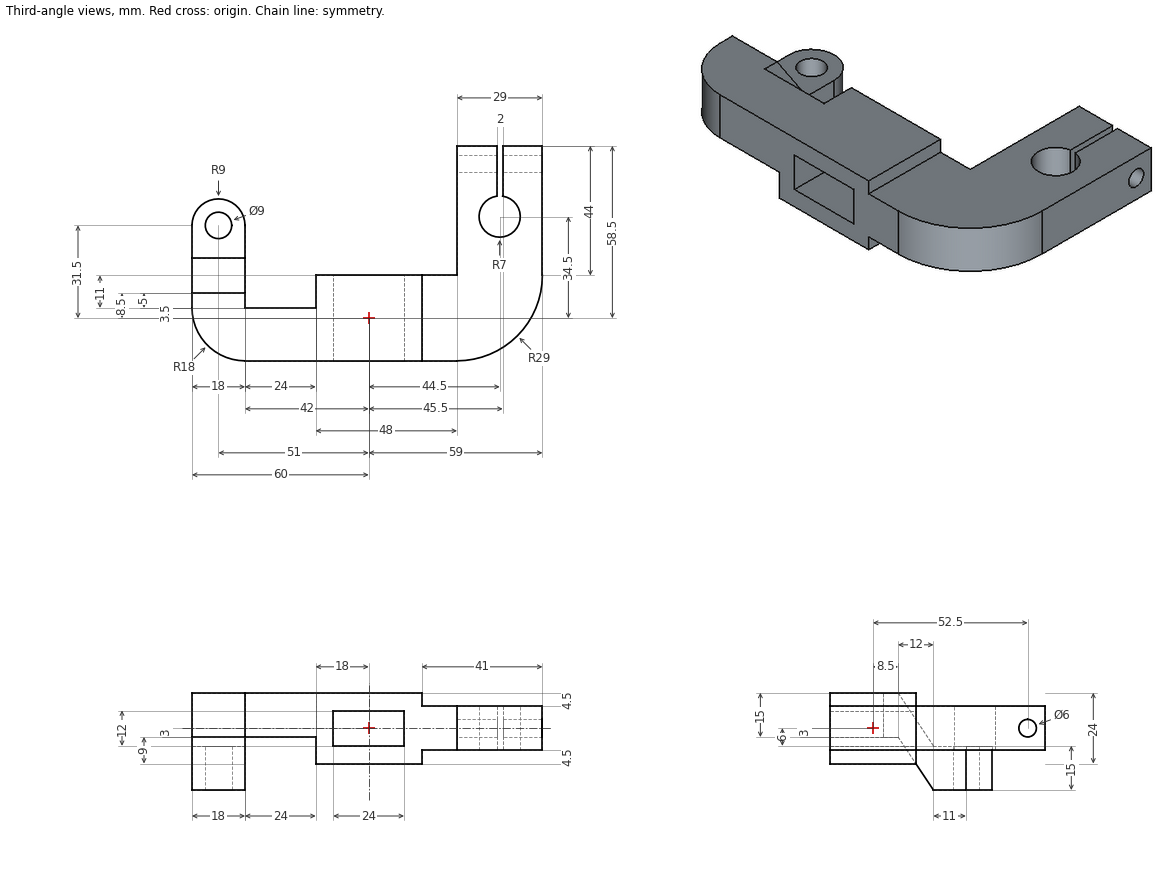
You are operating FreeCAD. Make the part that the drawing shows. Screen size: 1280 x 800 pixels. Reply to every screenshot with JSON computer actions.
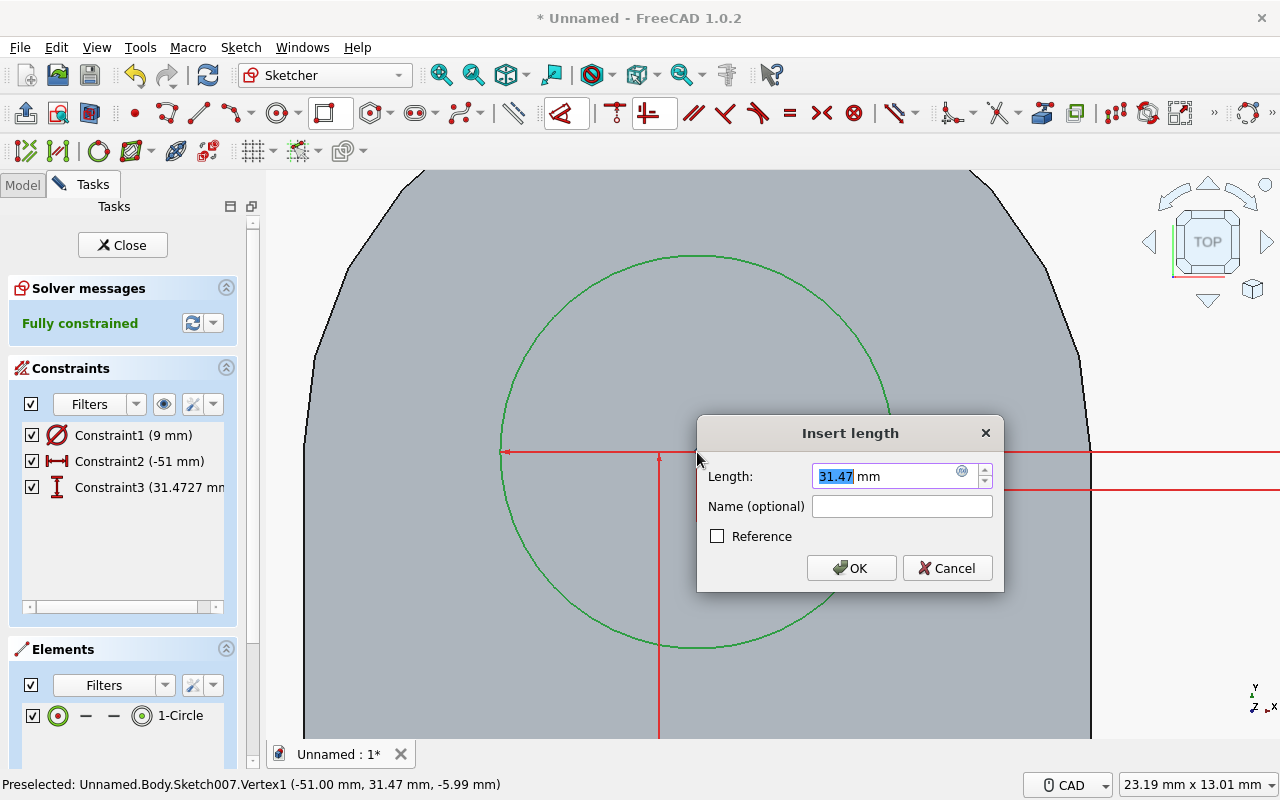
{"action": "type", "text": "31.5"}
{"action": "key", "text": "Return"}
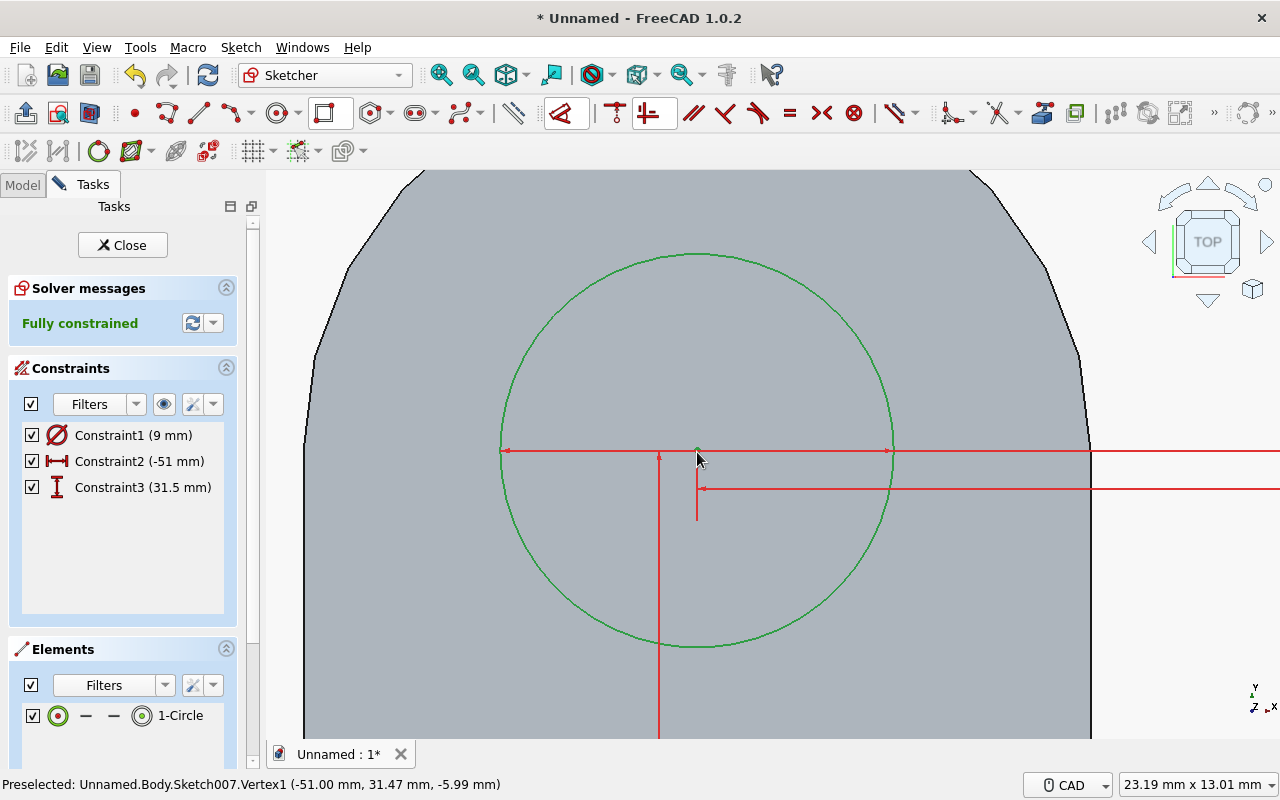
{"action": "left_click", "coordinate": [123, 245]}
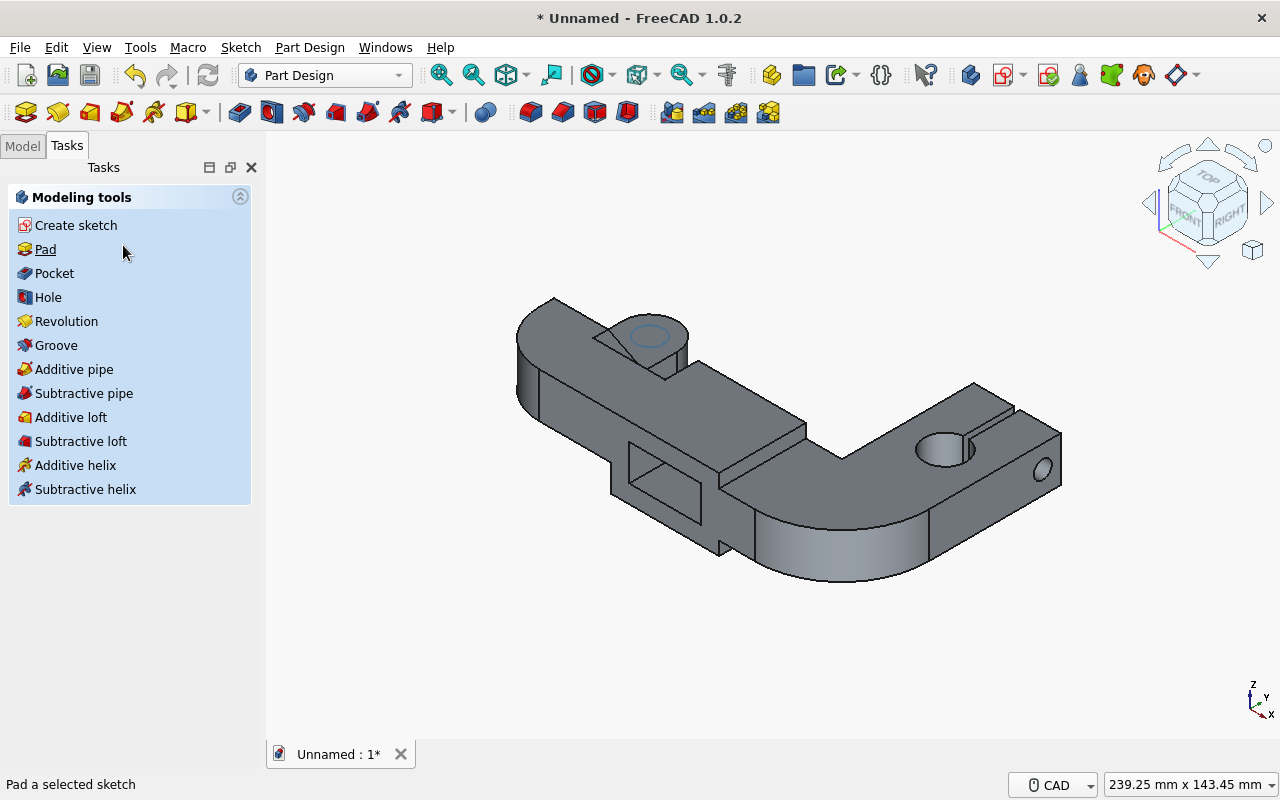
{"action": "left_click", "coordinate": [240, 112]}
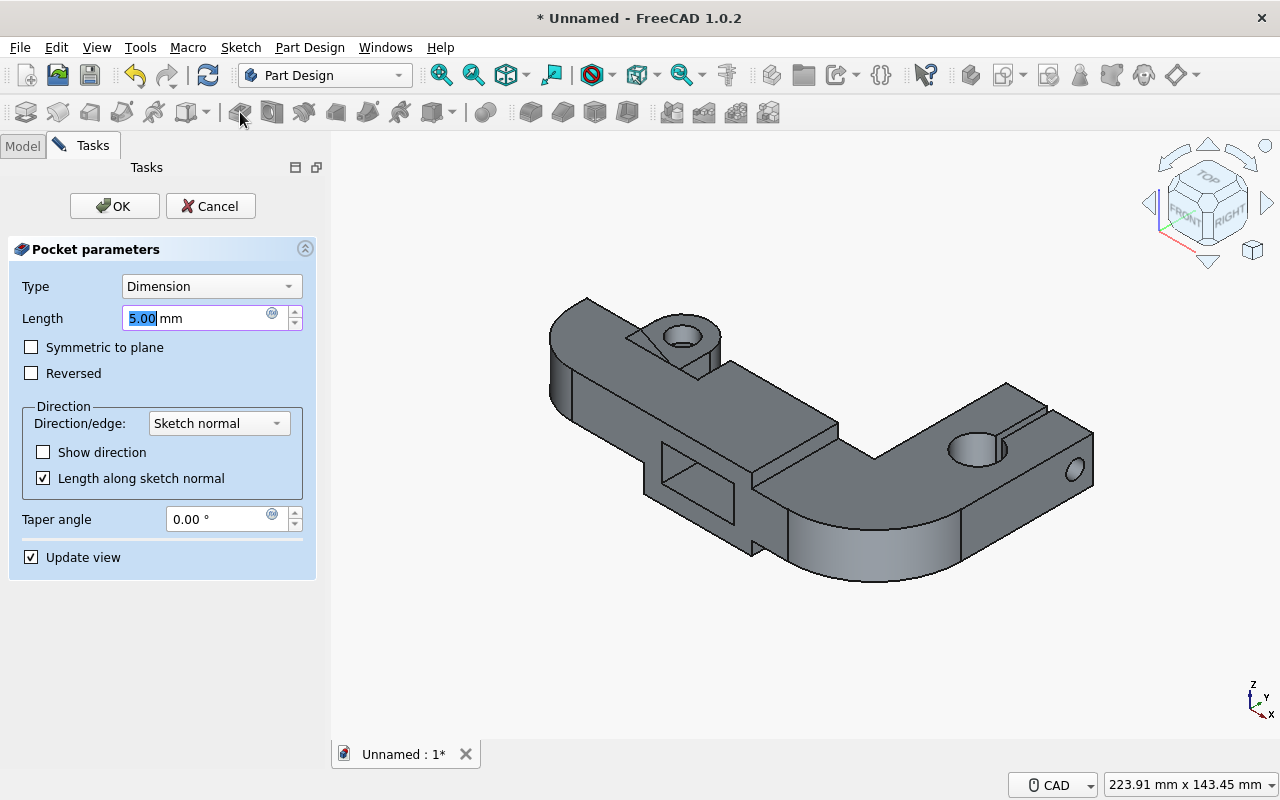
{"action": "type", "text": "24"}
{"action": "key", "text": "Tab"}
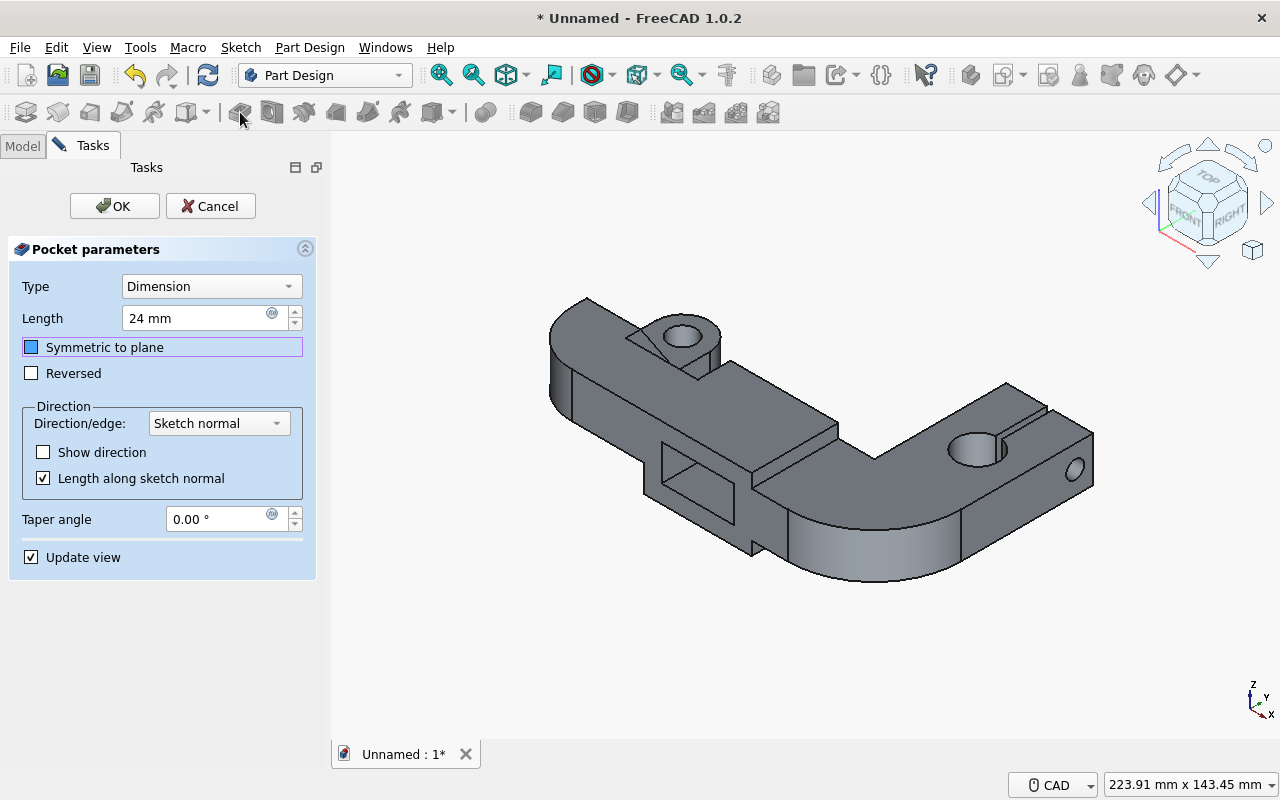
{"action": "left_click", "coordinate": [115, 206]}